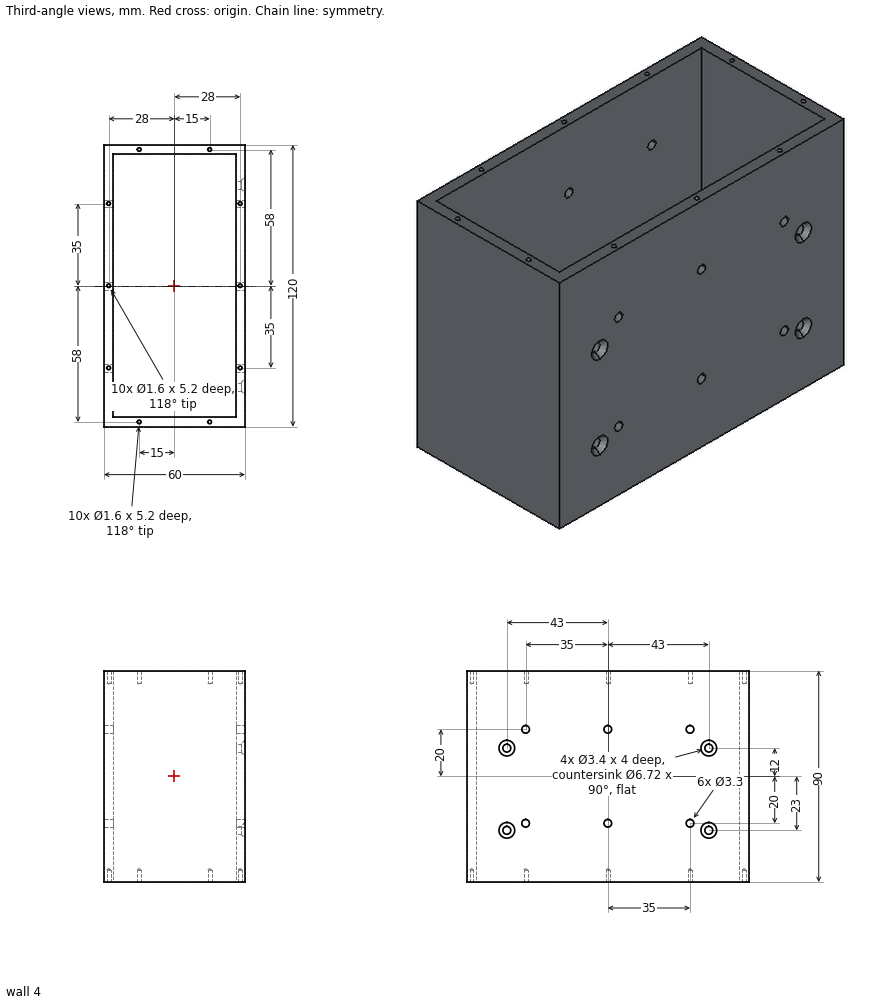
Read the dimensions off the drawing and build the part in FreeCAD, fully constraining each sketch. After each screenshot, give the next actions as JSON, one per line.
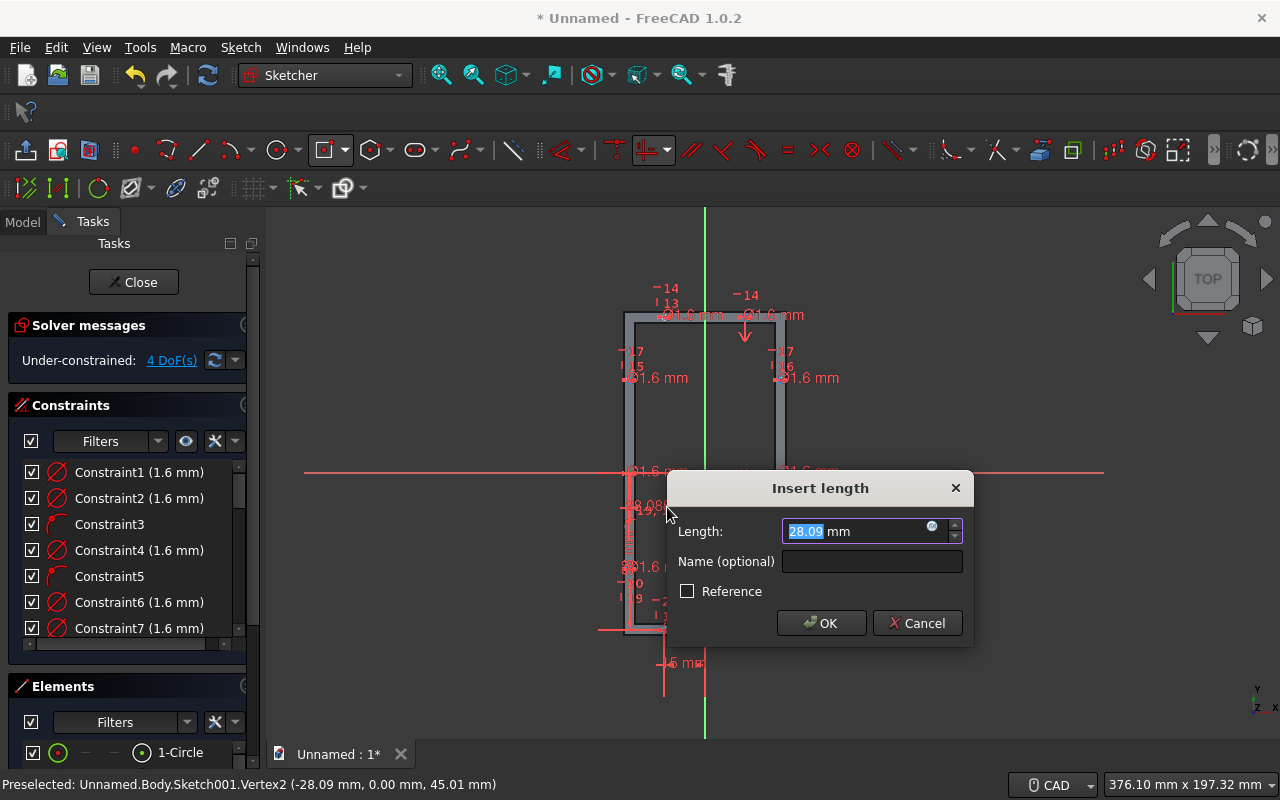
{"action": "type", "text": "28"}
{"action": "key", "text": "Return"}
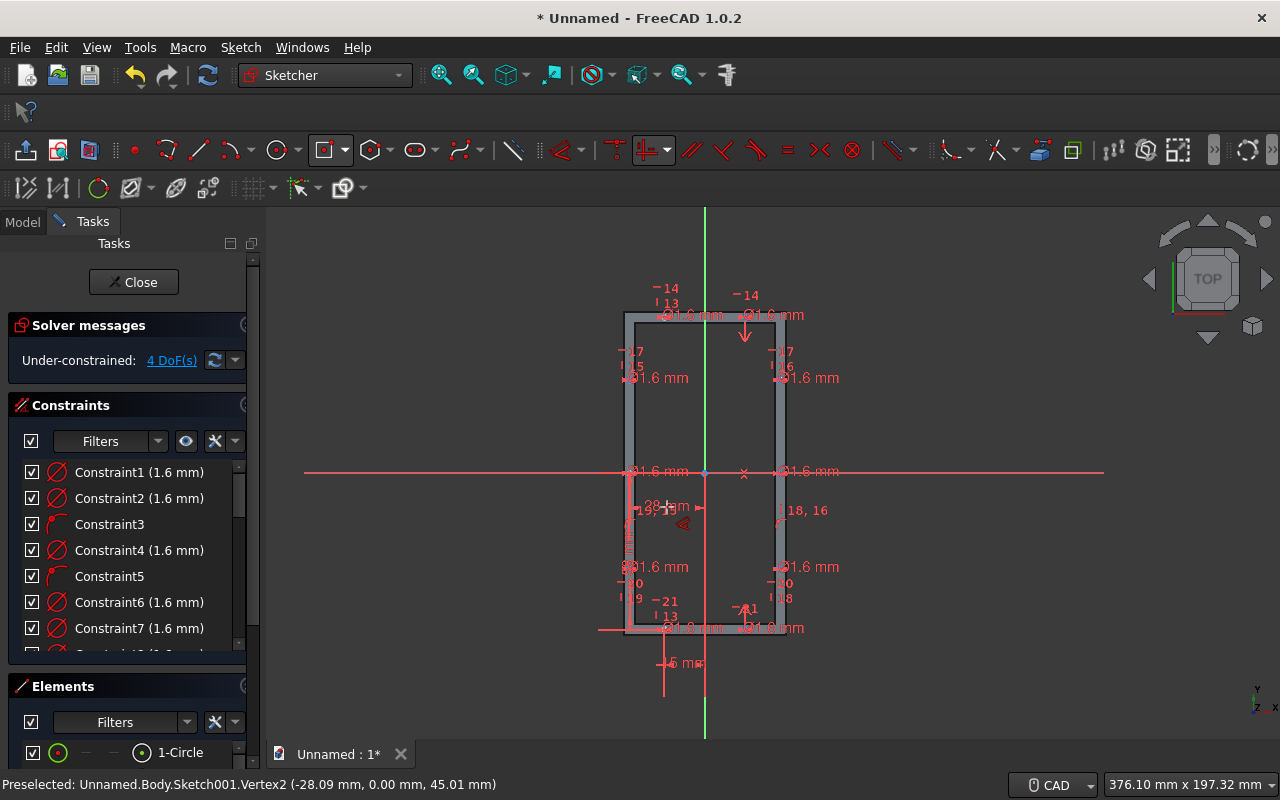
{"action": "left_click", "coordinate": [780, 473]}
{"action": "left_click", "coordinate": [742, 507]}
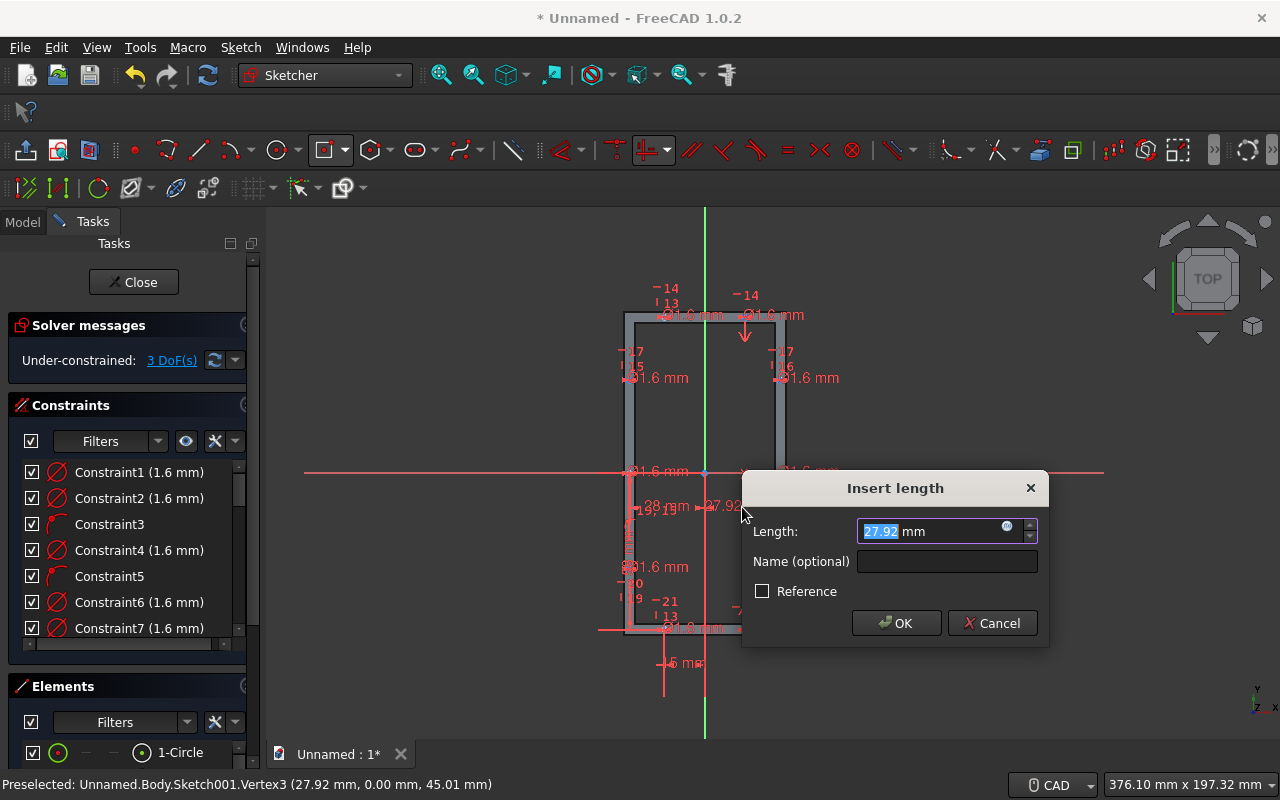
{"action": "type", "text": "28"}
{"action": "key", "text": "Return"}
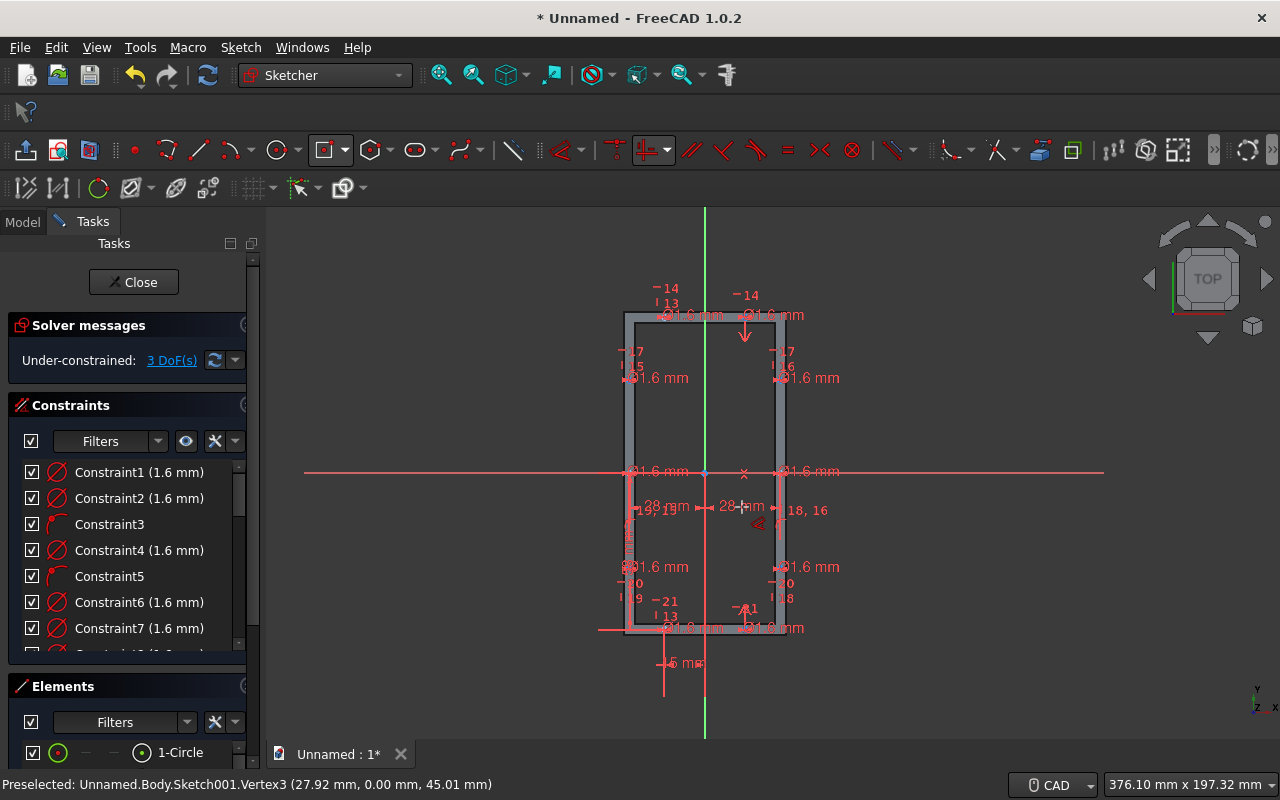
{"action": "left_click", "coordinate": [745, 317]}
{"action": "left_click", "coordinate": [725, 283]}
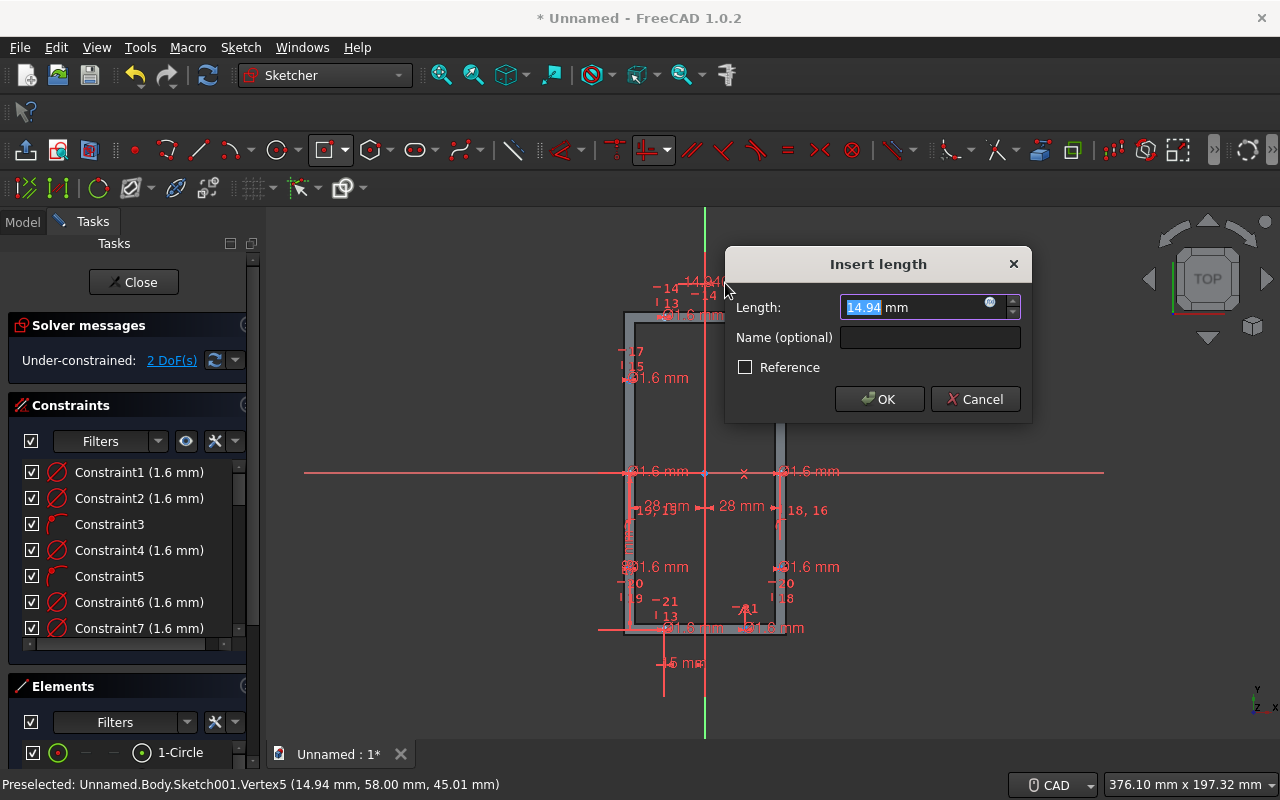
{"action": "type", "text": "15"}
{"action": "key", "text": "Return"}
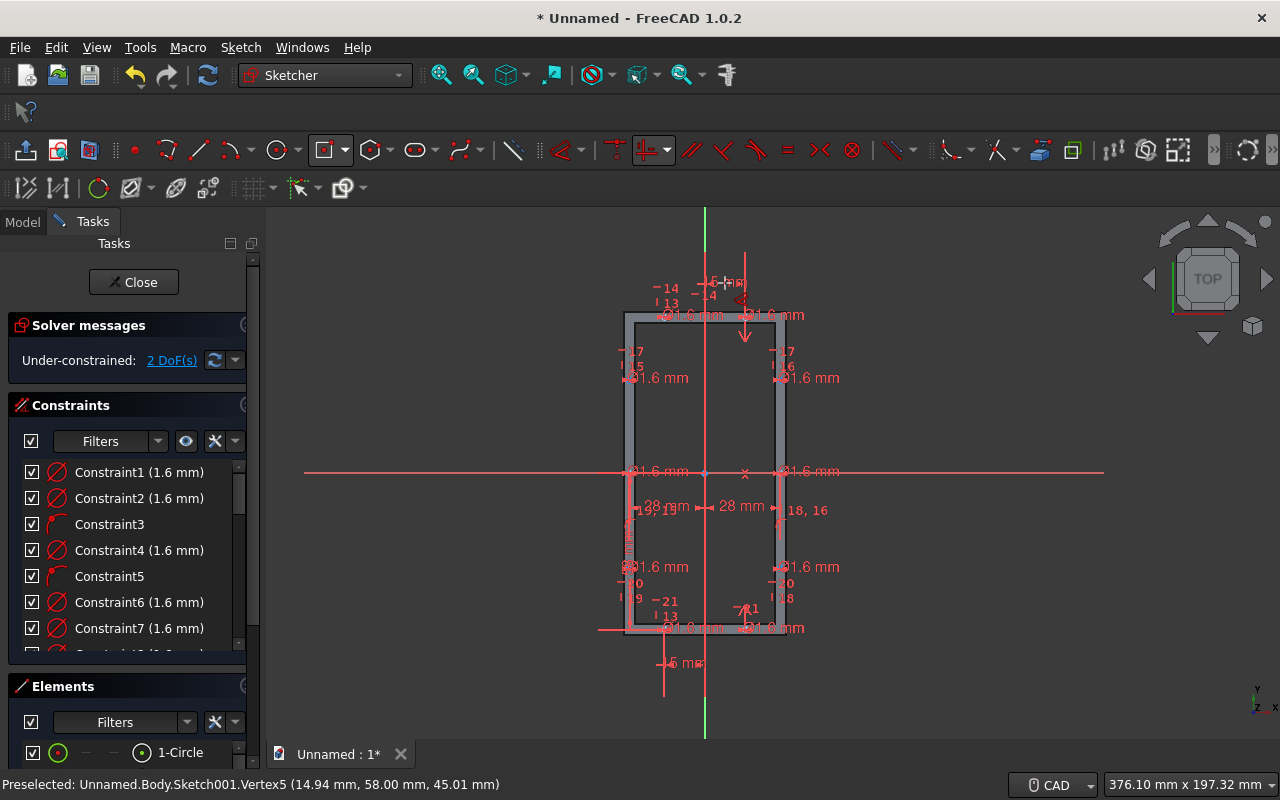
{"action": "left_click", "coordinate": [629, 380]}
{"action": "left_click", "coordinate": [595, 427]}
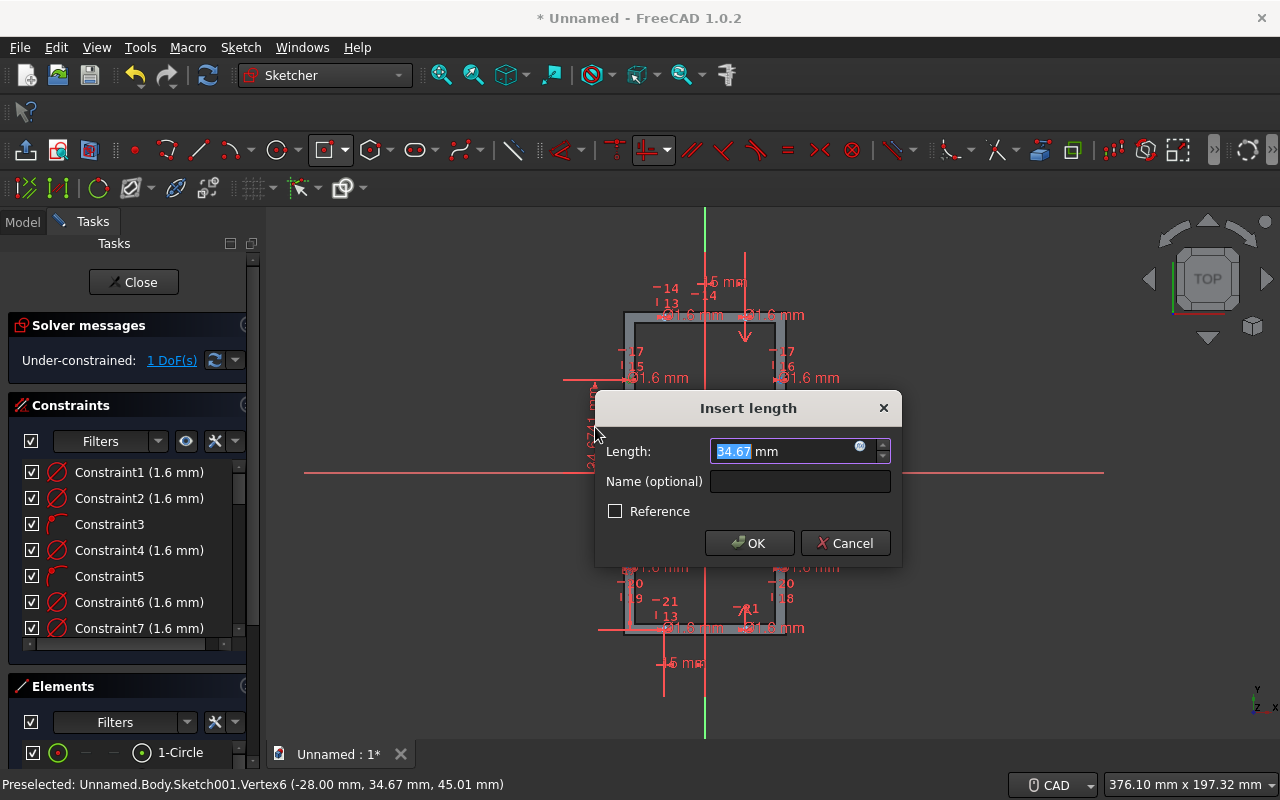
{"action": "type", "text": "35"}
{"action": "key", "text": "Return"}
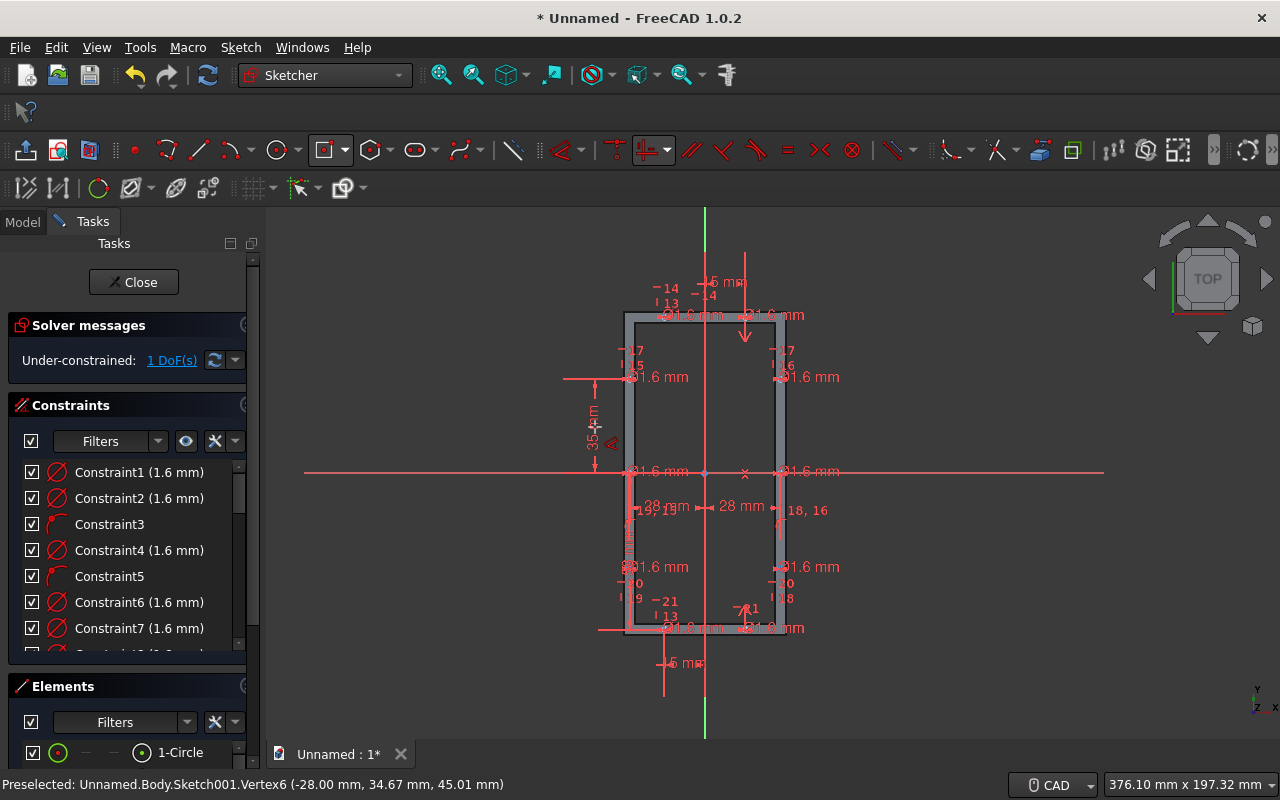
{"action": "left_click", "coordinate": [780, 569]}
{"action": "left_click", "coordinate": [814, 521]}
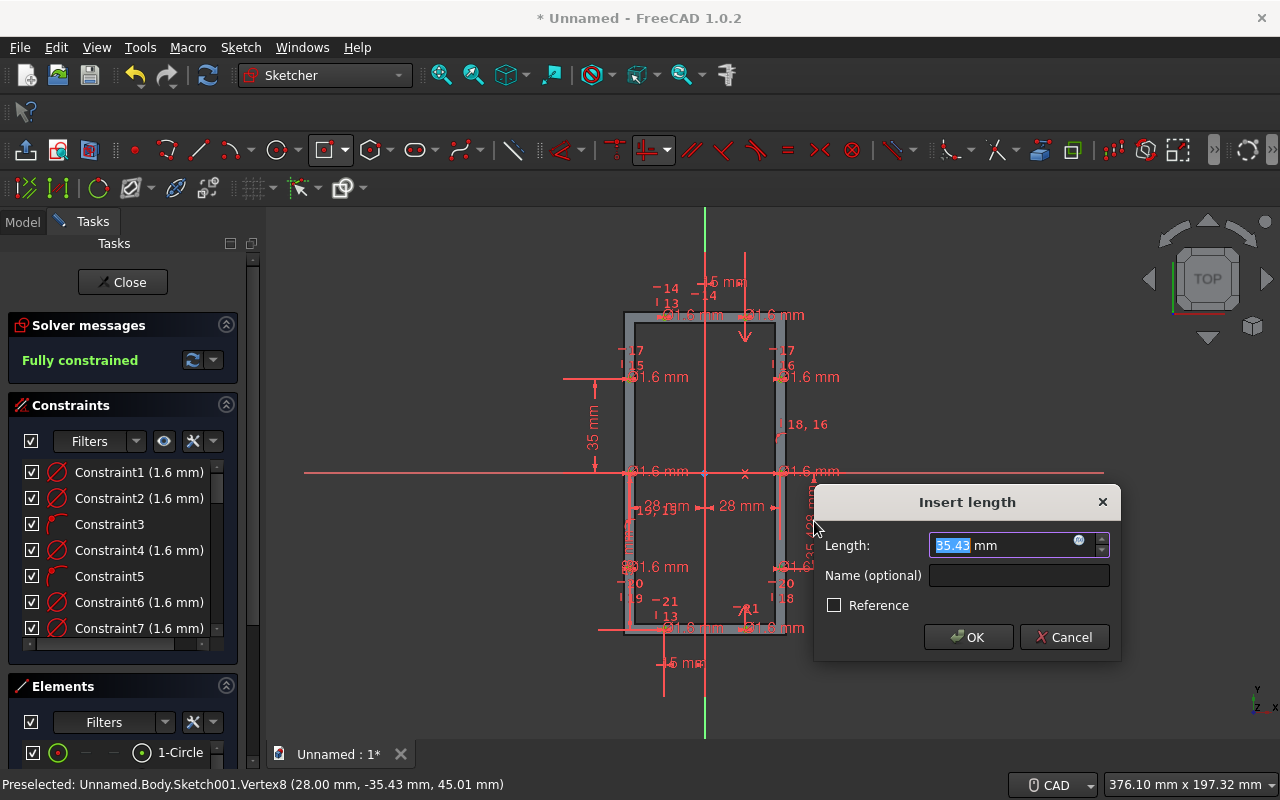
{"action": "type", "text": "35"}
{"action": "key", "text": "Return"}
{"action": "key", "text": "Escape"}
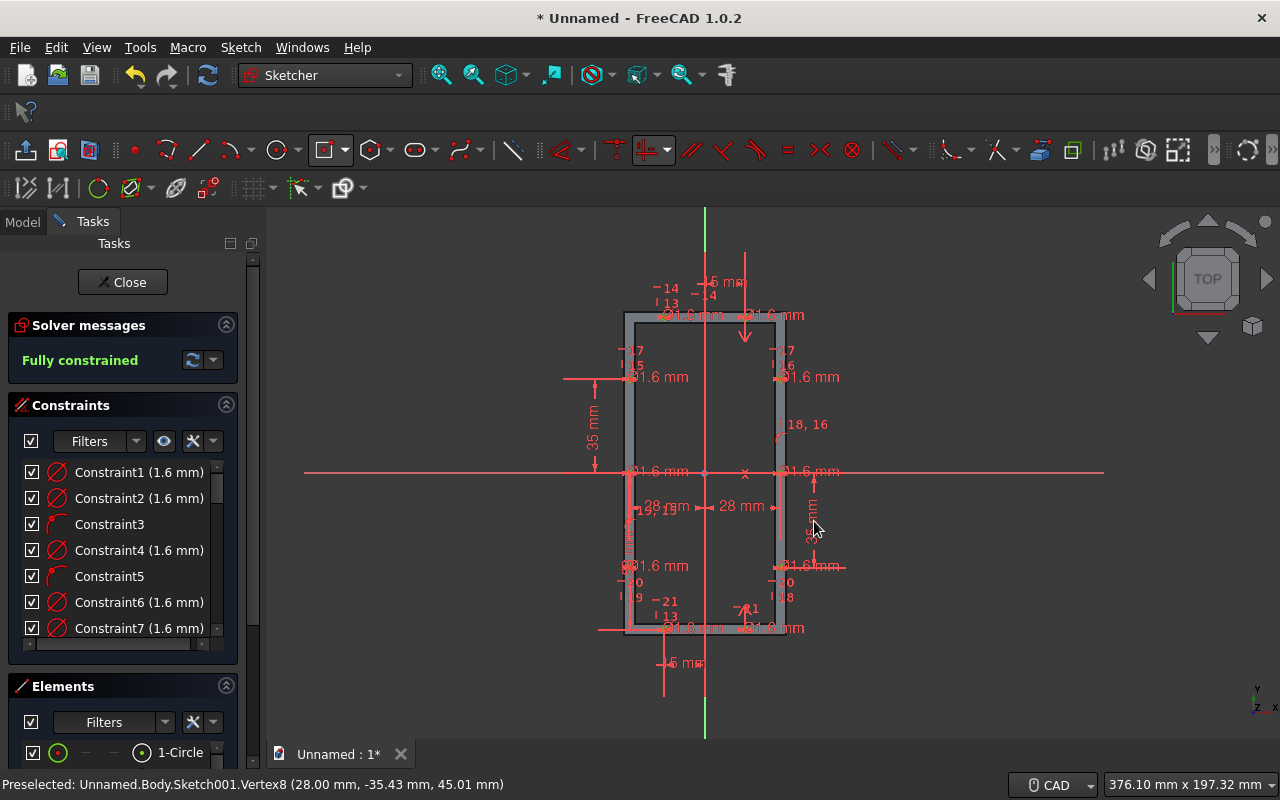
{"action": "left_click", "coordinate": [123, 282]}